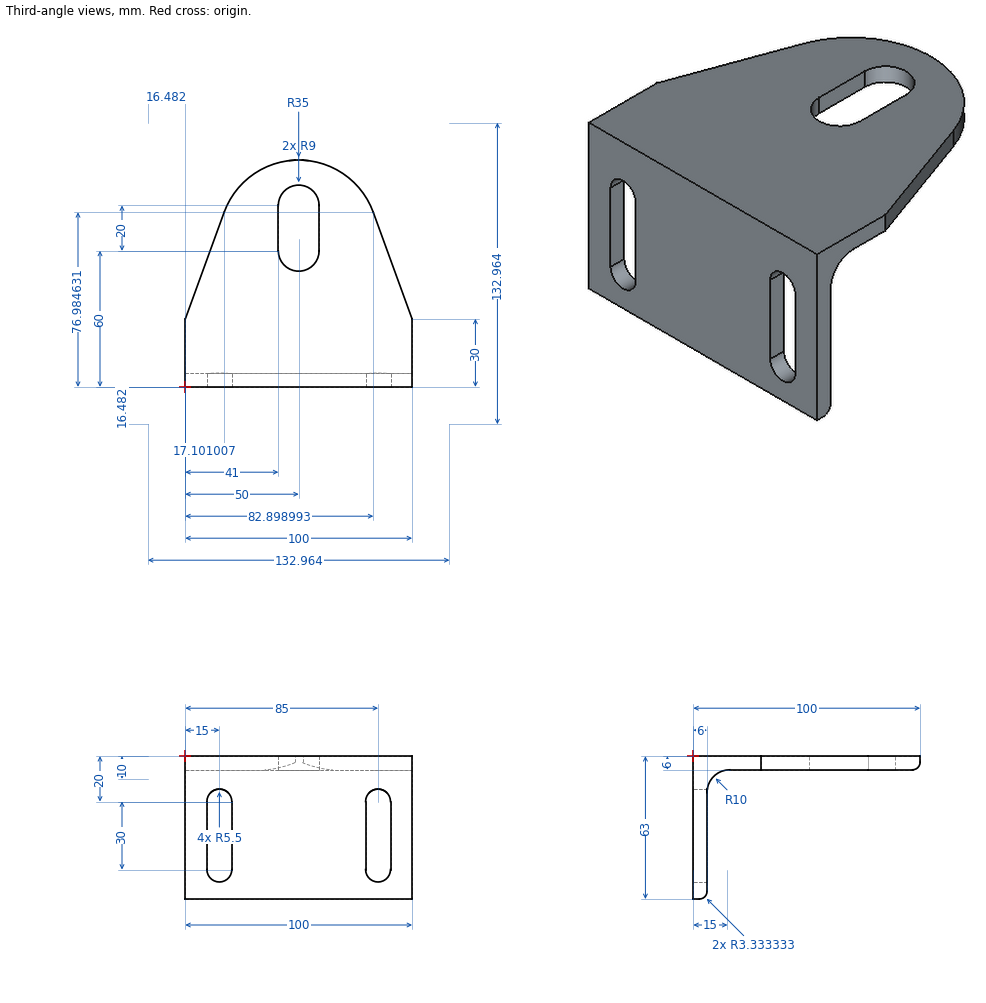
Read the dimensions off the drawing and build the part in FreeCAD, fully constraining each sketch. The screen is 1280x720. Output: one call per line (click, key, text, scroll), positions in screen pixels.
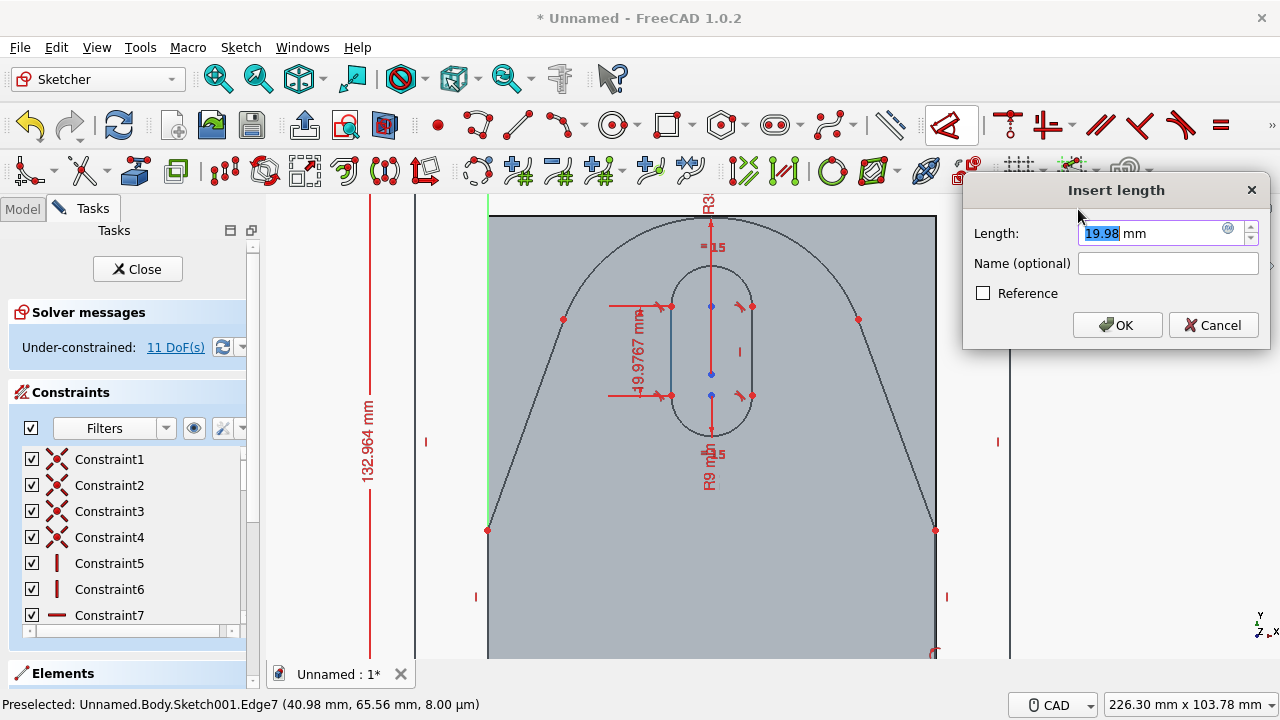
text(20)
key(Return)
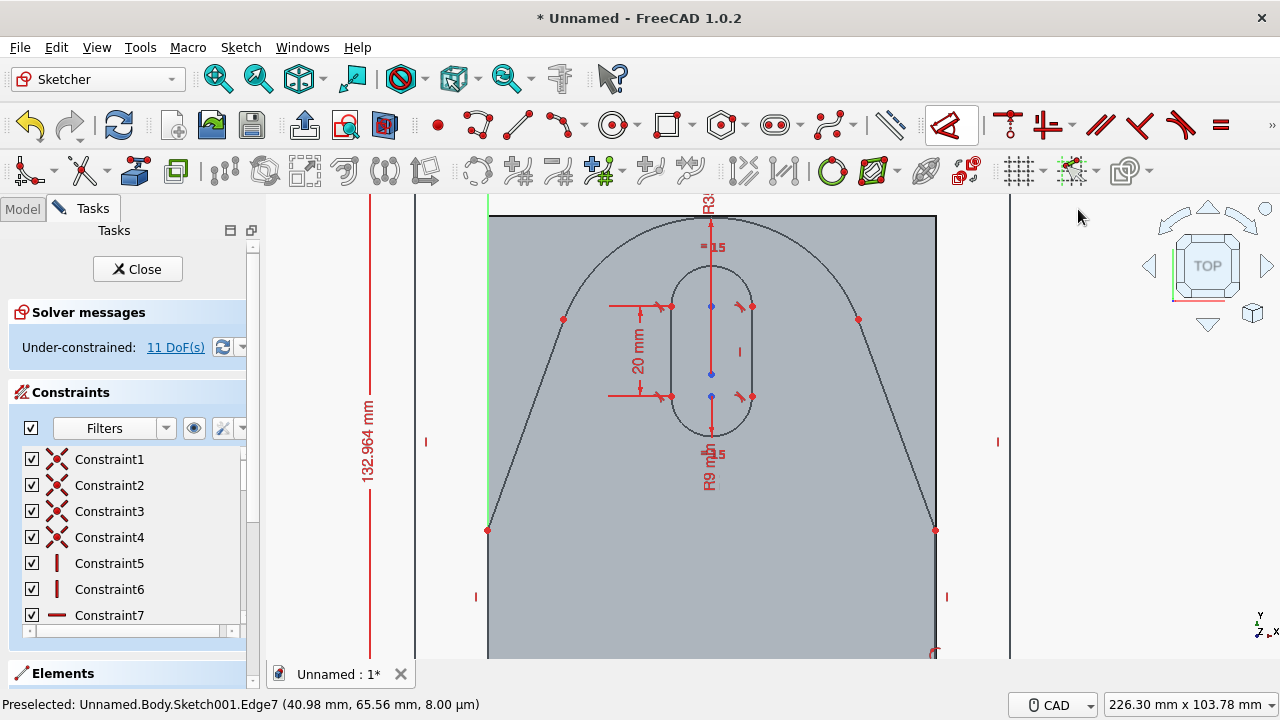
click(935, 570)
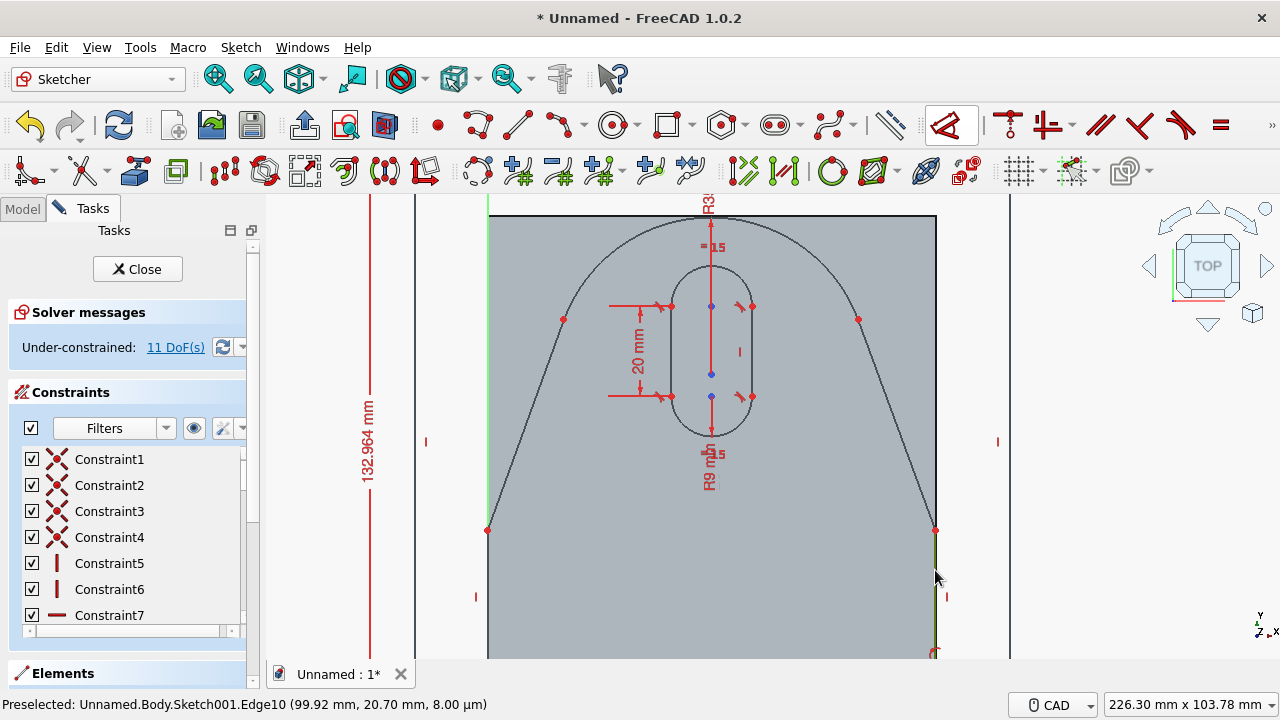
click(972, 126)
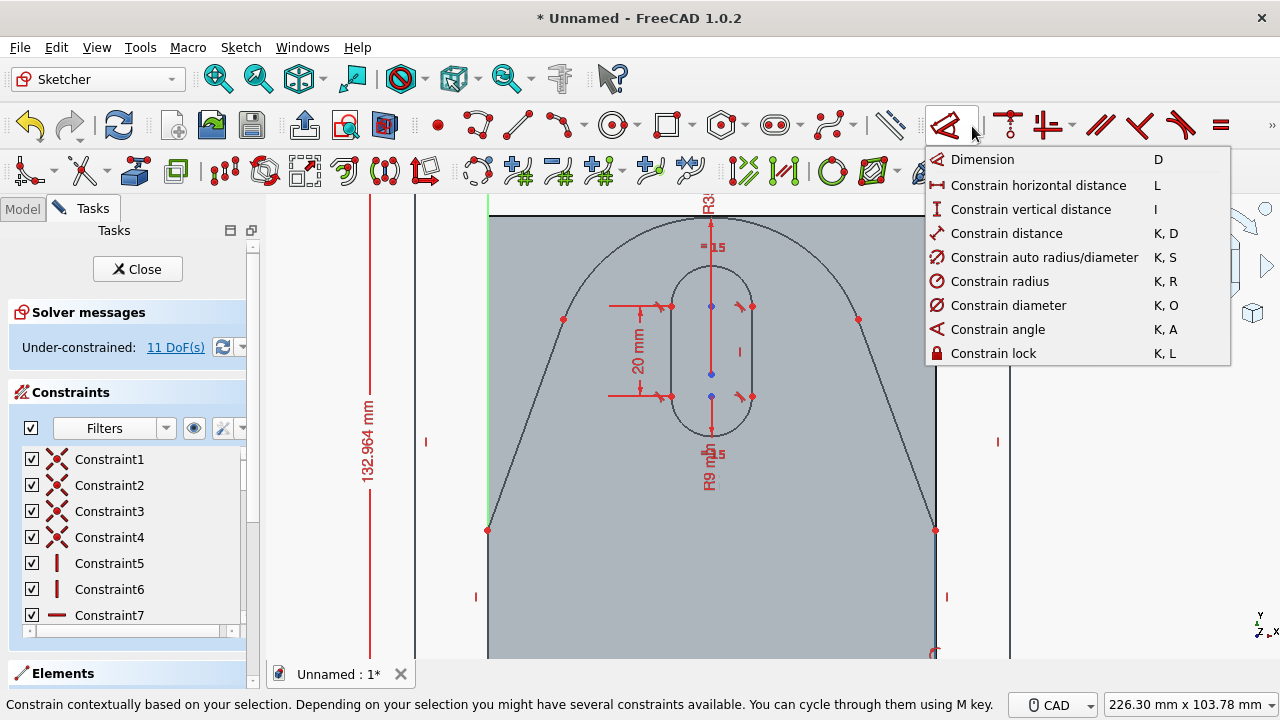
click(1078, 209)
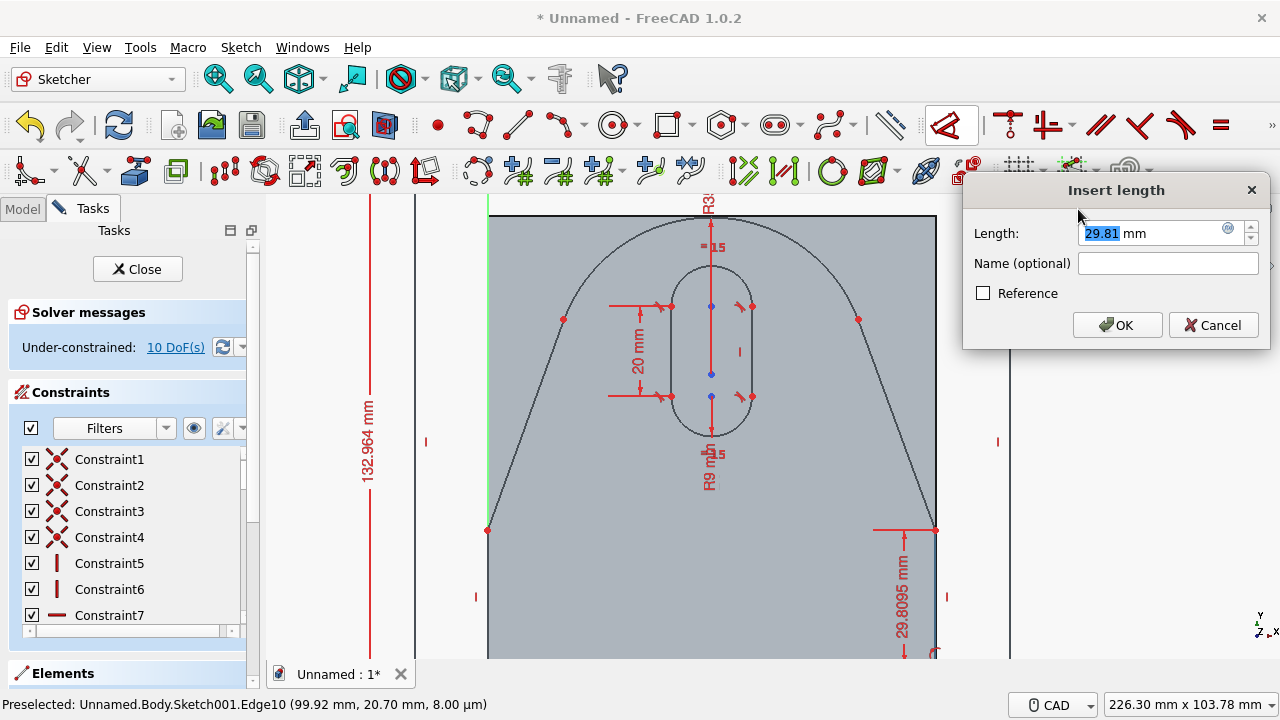
text(30)
key(Return)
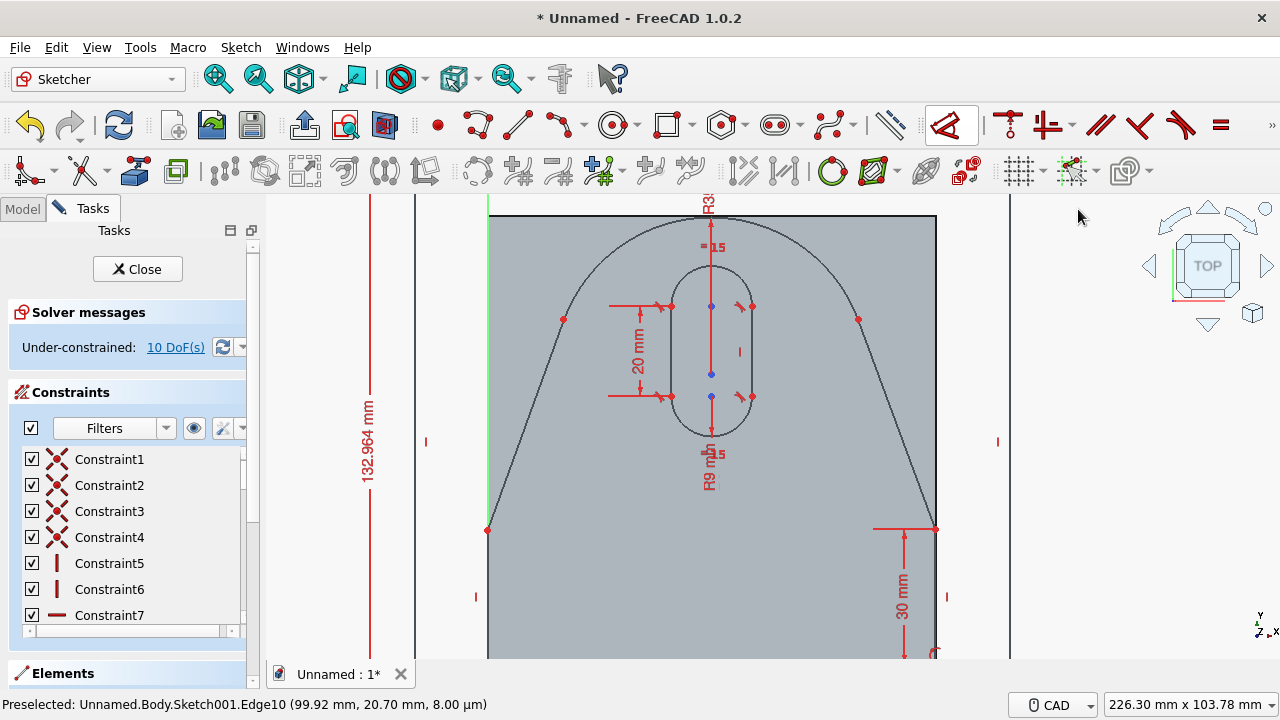
click(488, 624)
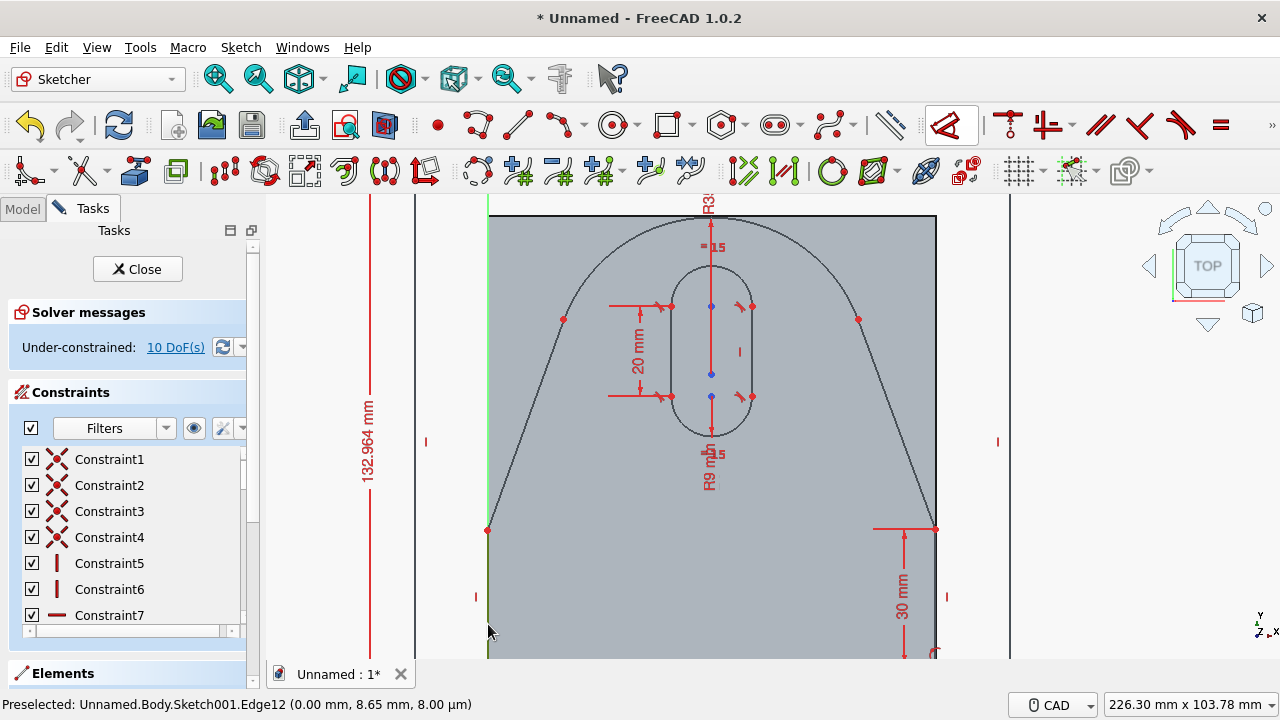
click(972, 126)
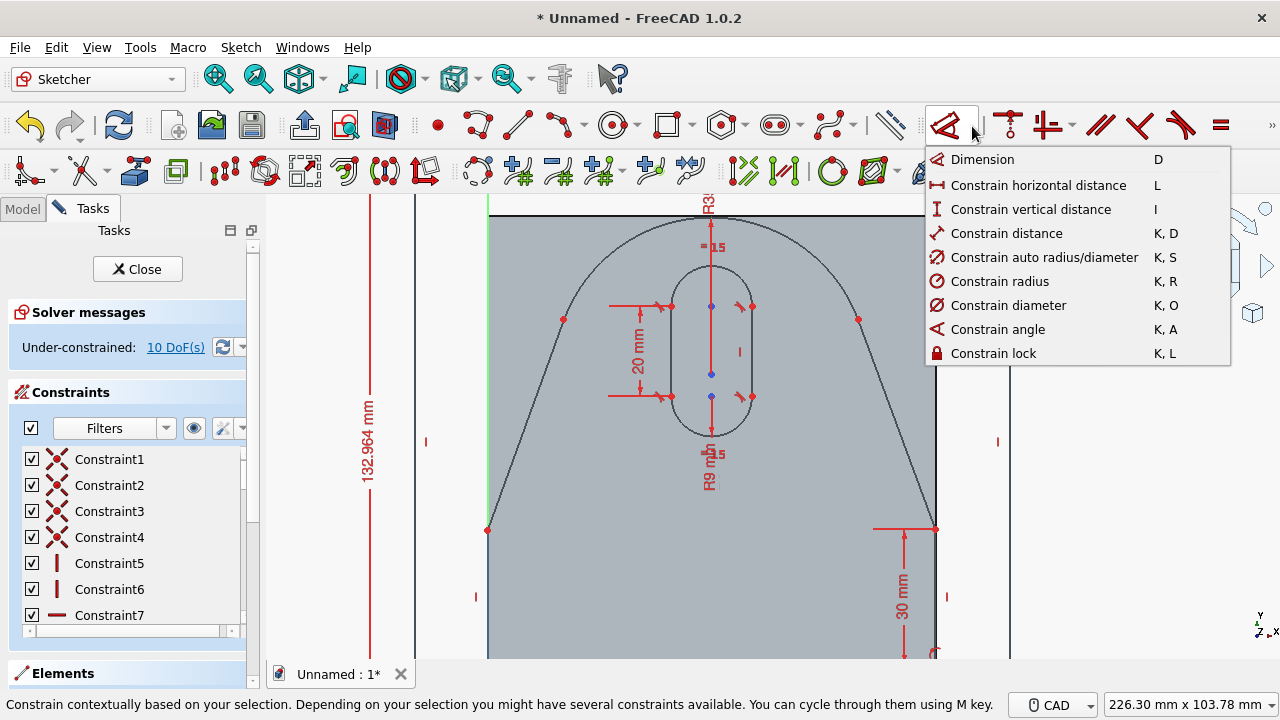
click(1078, 209)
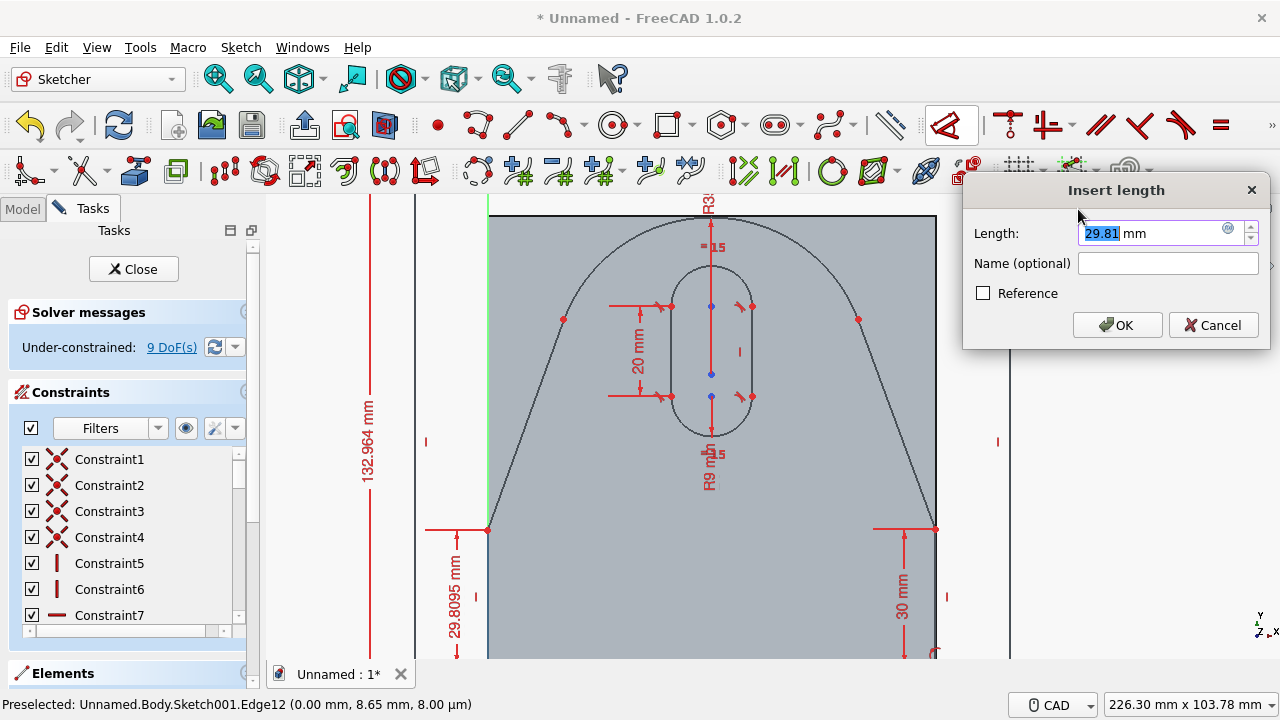
text(30)
key(Return)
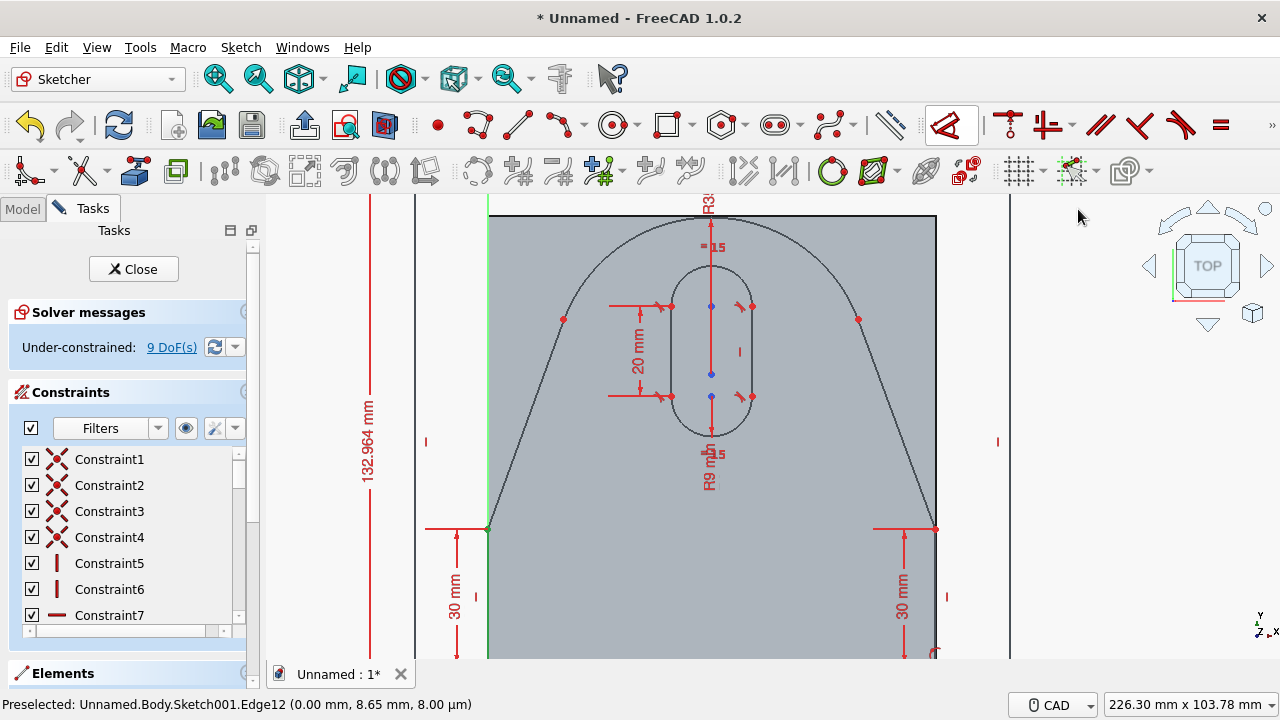
scroll(699, 416, down, 4)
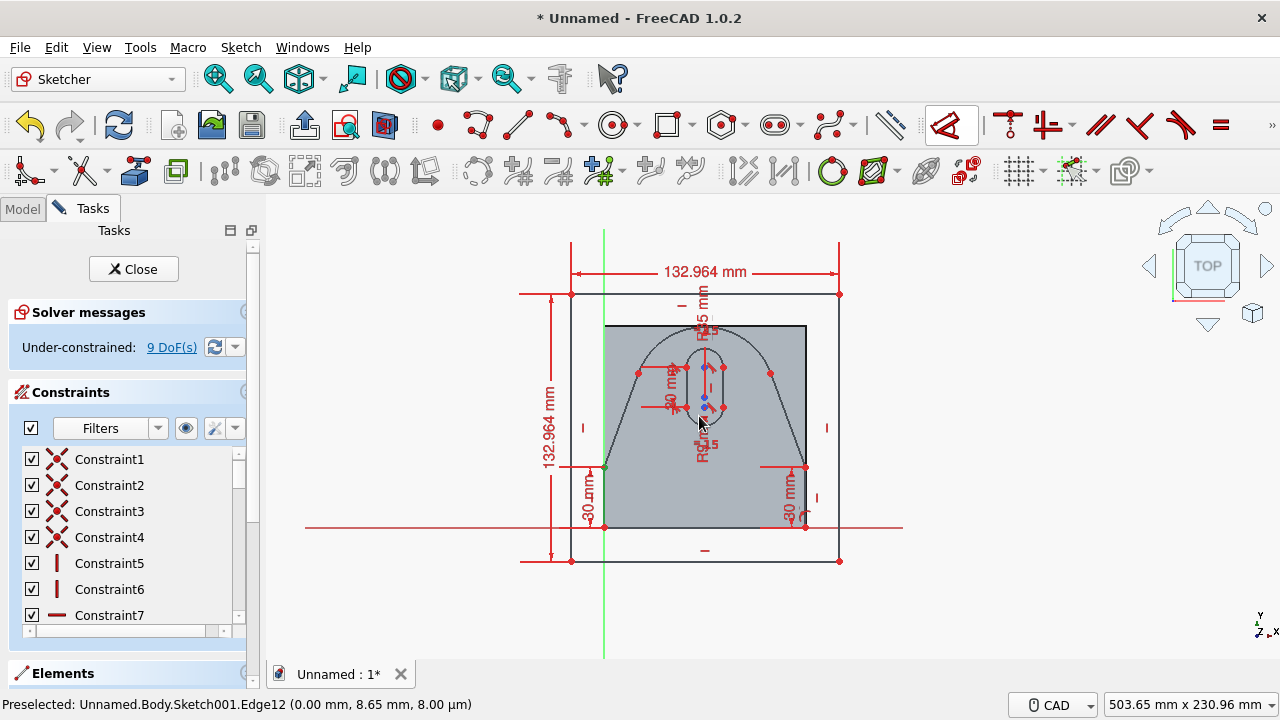
click(745, 528)